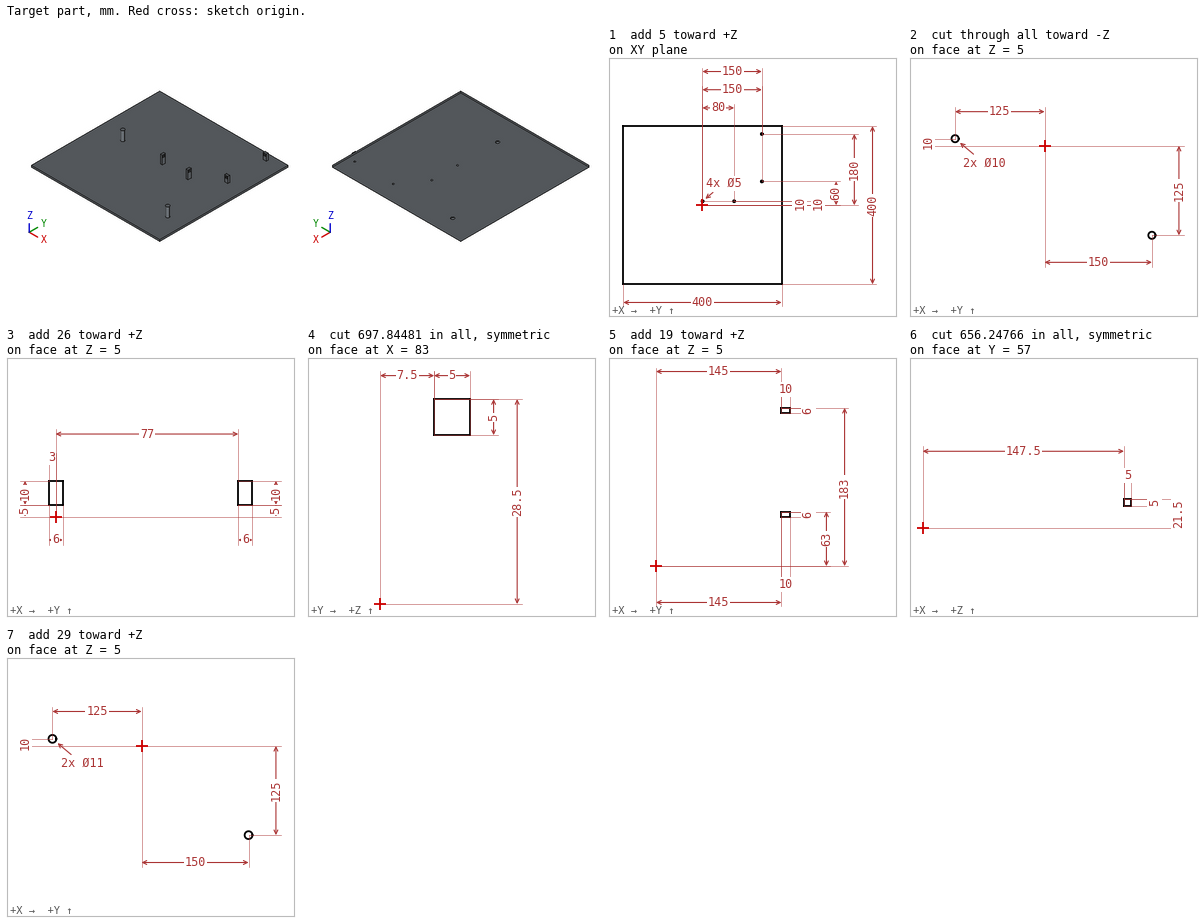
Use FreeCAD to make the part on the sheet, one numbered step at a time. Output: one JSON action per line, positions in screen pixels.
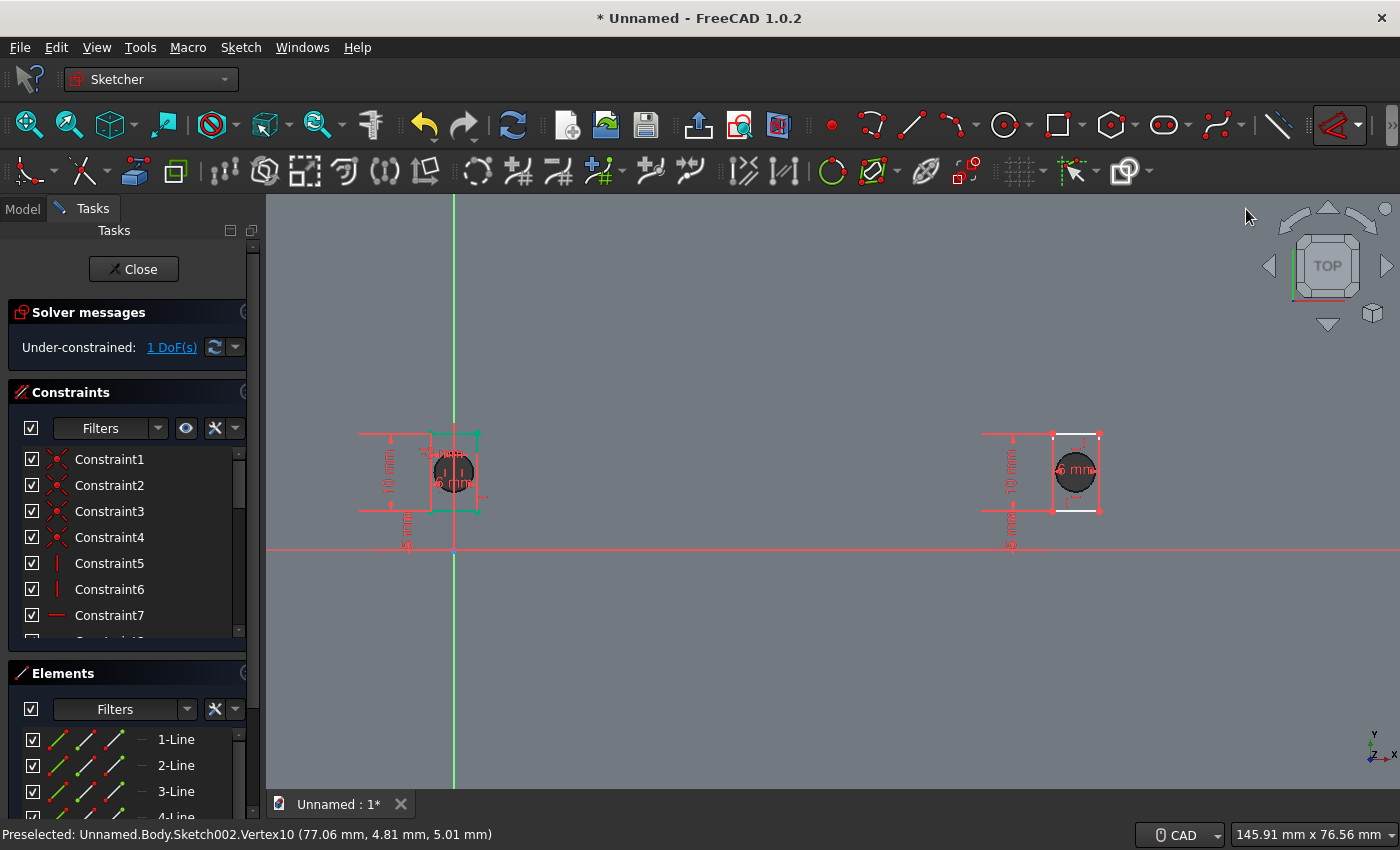
{"action": "left_click", "coordinate": [1053, 434]}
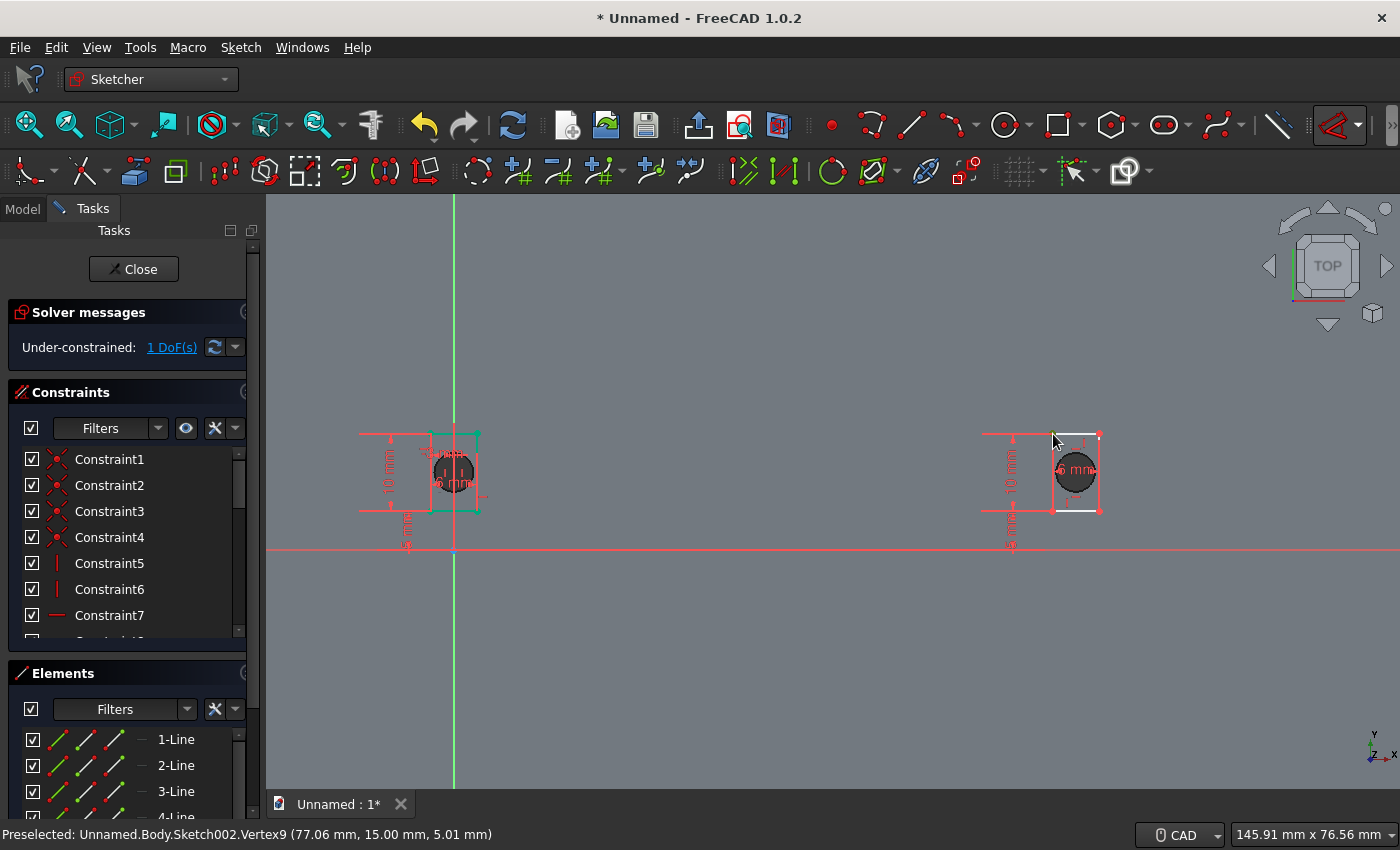
{"action": "key", "text": "l"}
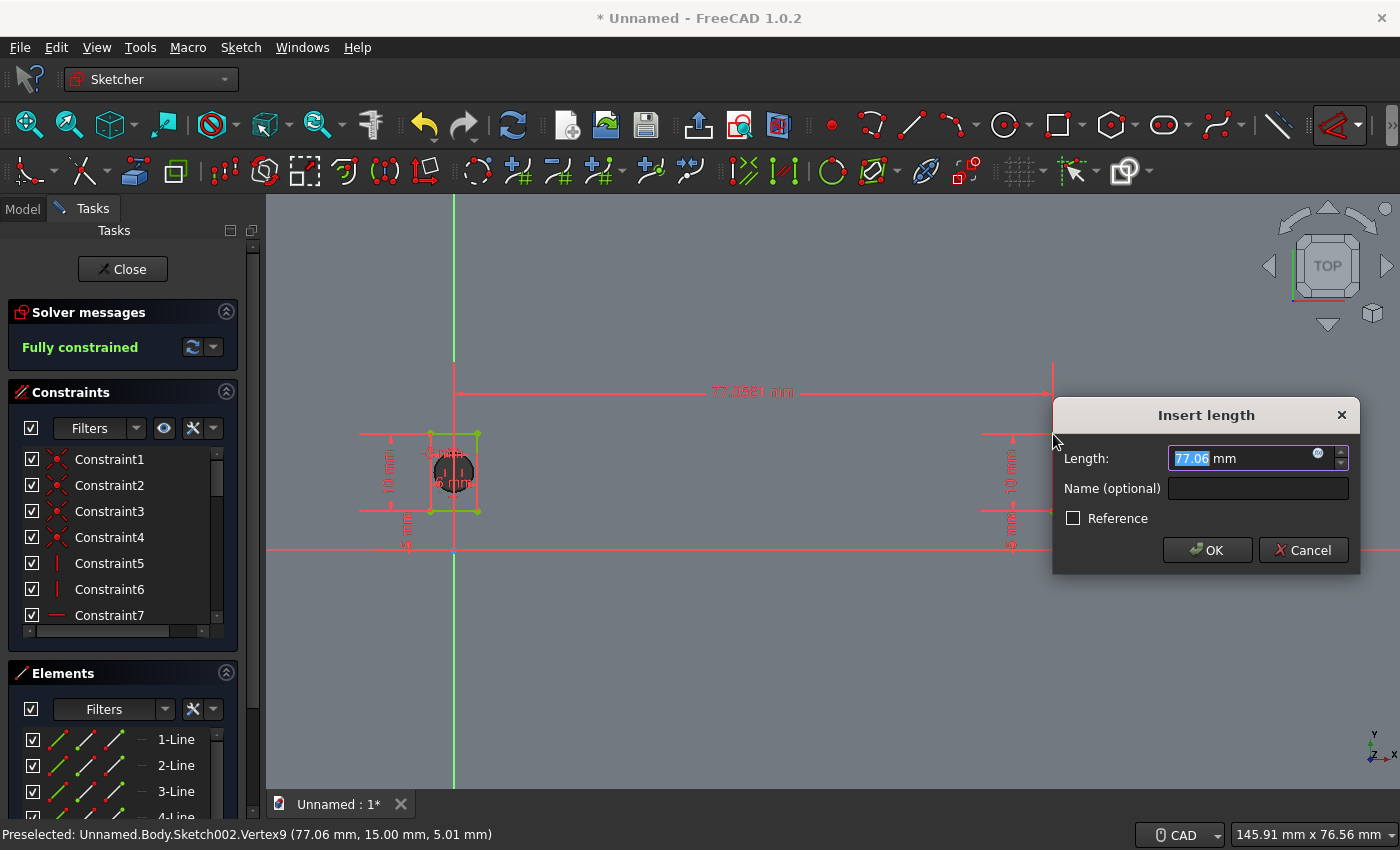
{"action": "type", "text": "77"}
{"action": "key", "text": "Return"}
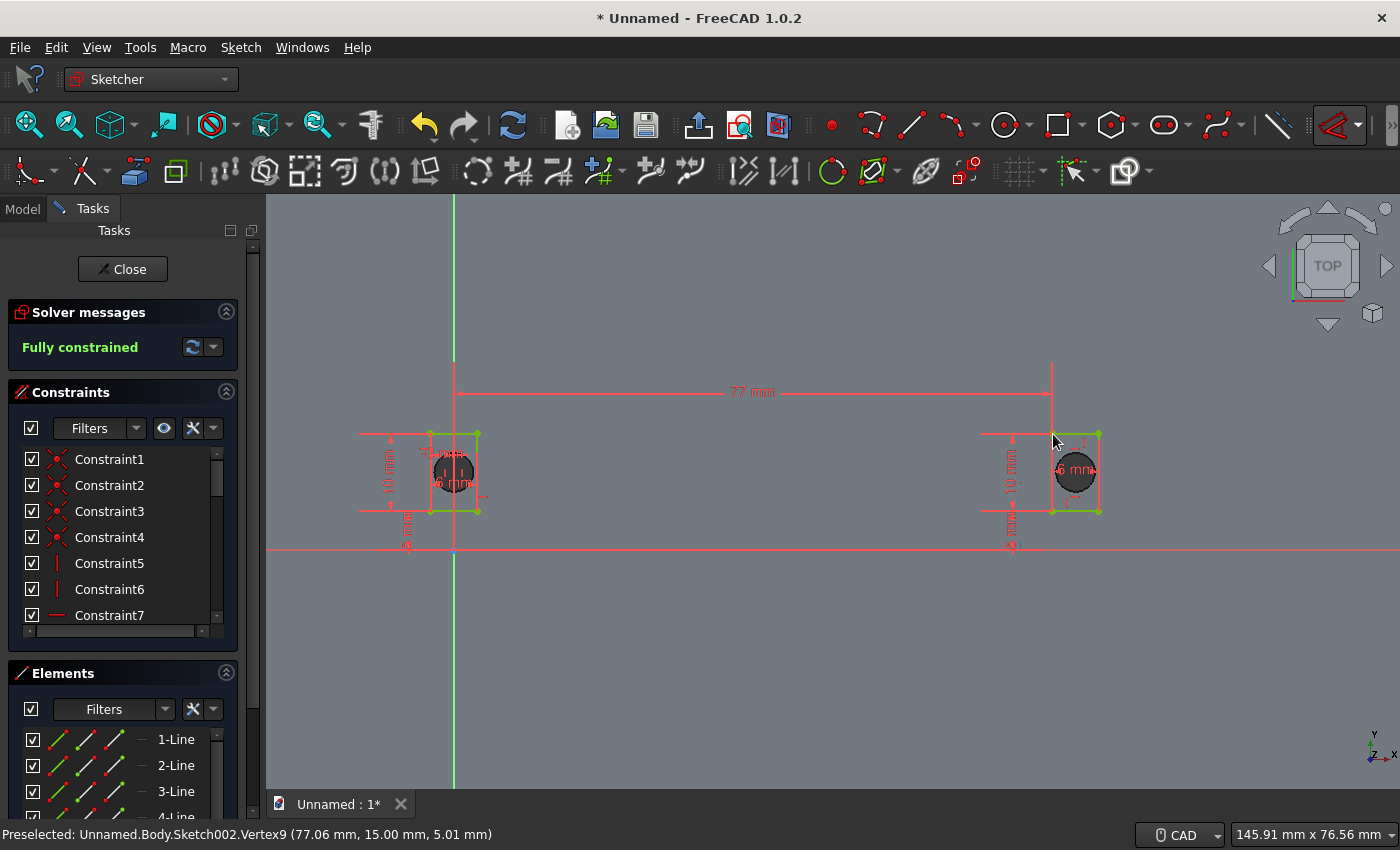
{"action": "left_click", "coordinate": [123, 269]}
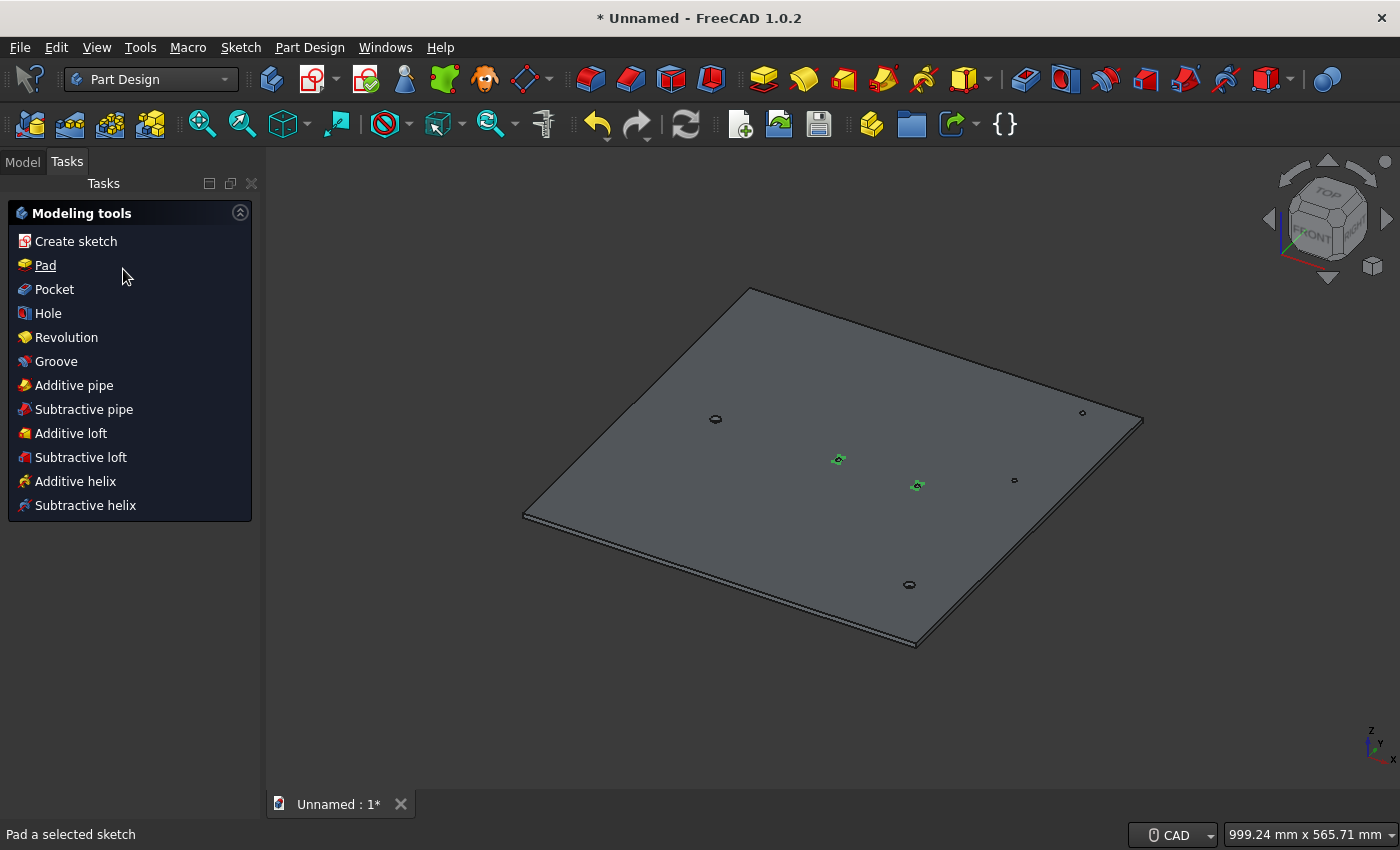
{"action": "left_click", "coordinate": [764, 80]}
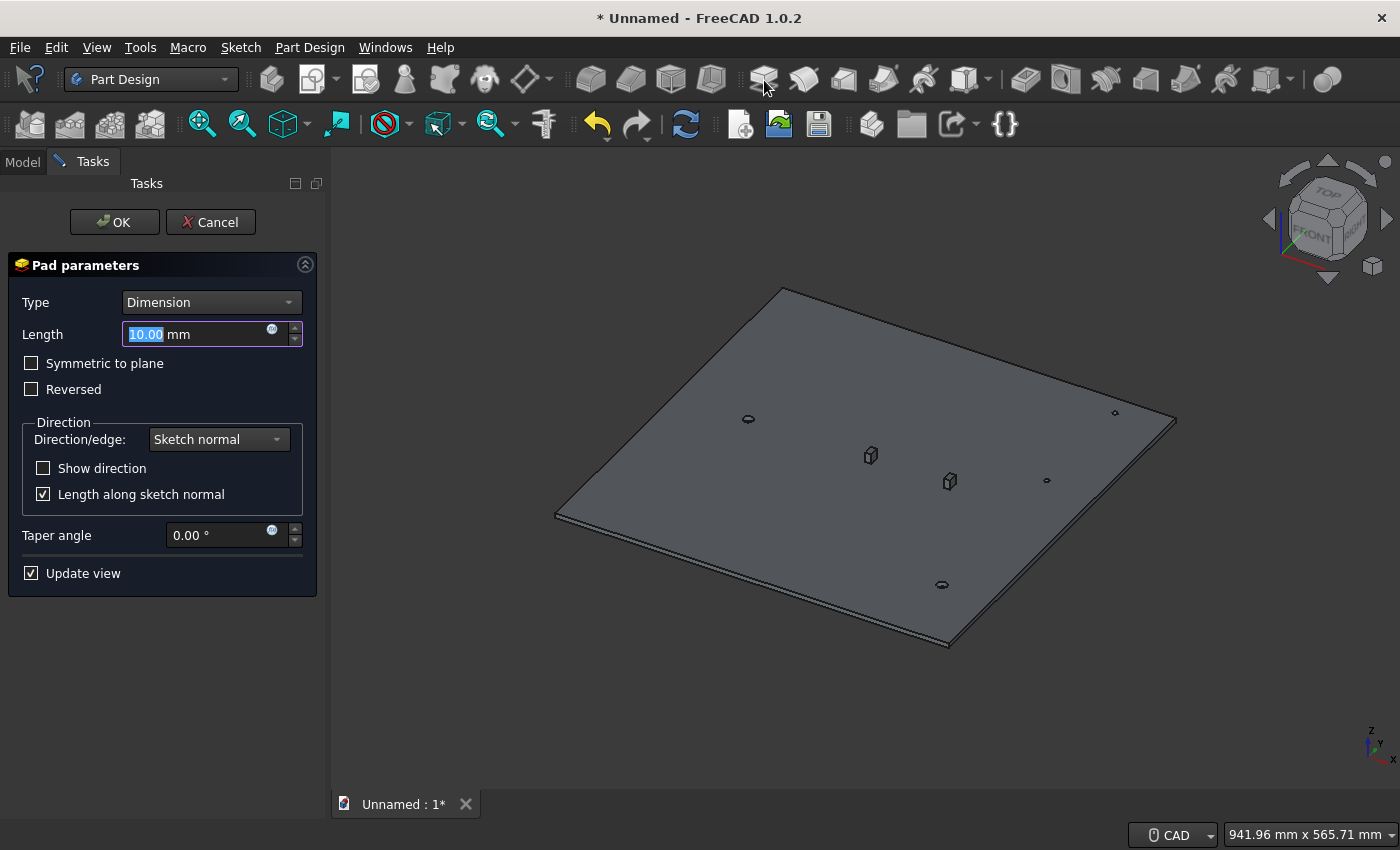
{"action": "type", "text": "26"}
{"action": "key", "text": "Tab"}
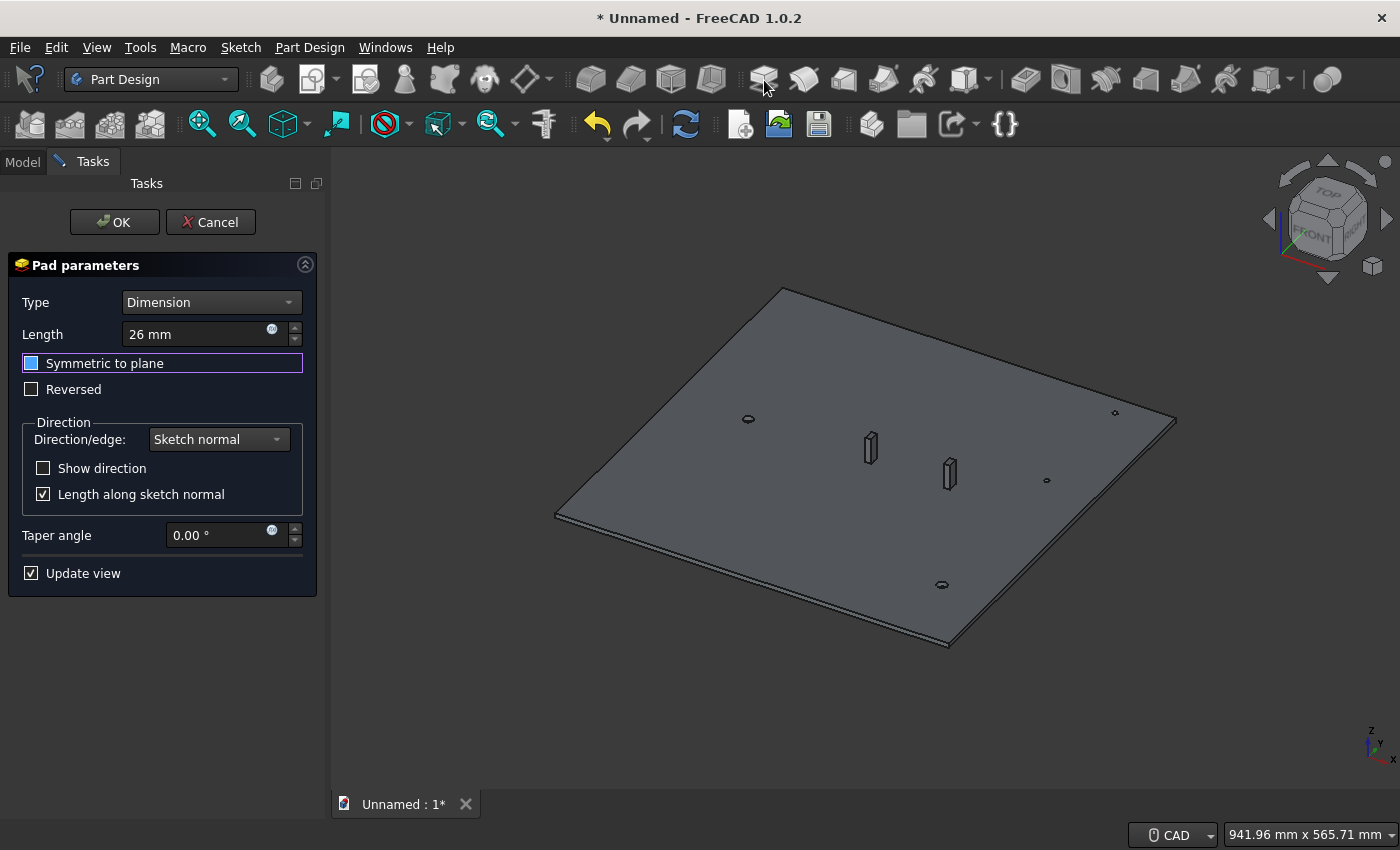
{"action": "left_click", "coordinate": [115, 222]}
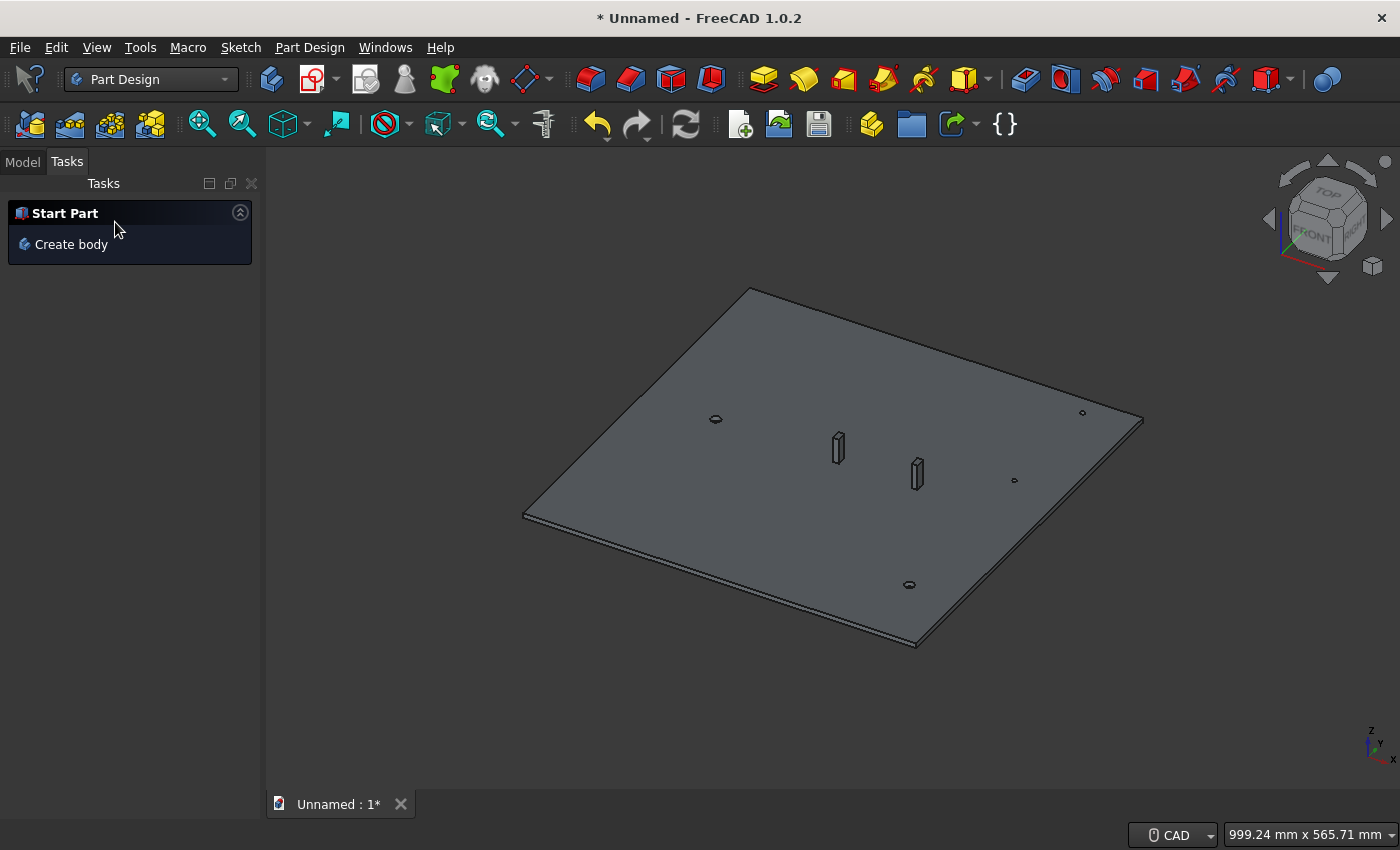
{"action": "scroll", "coordinate": [920, 467], "scroll_direction": "up", "scroll_amount": 4}